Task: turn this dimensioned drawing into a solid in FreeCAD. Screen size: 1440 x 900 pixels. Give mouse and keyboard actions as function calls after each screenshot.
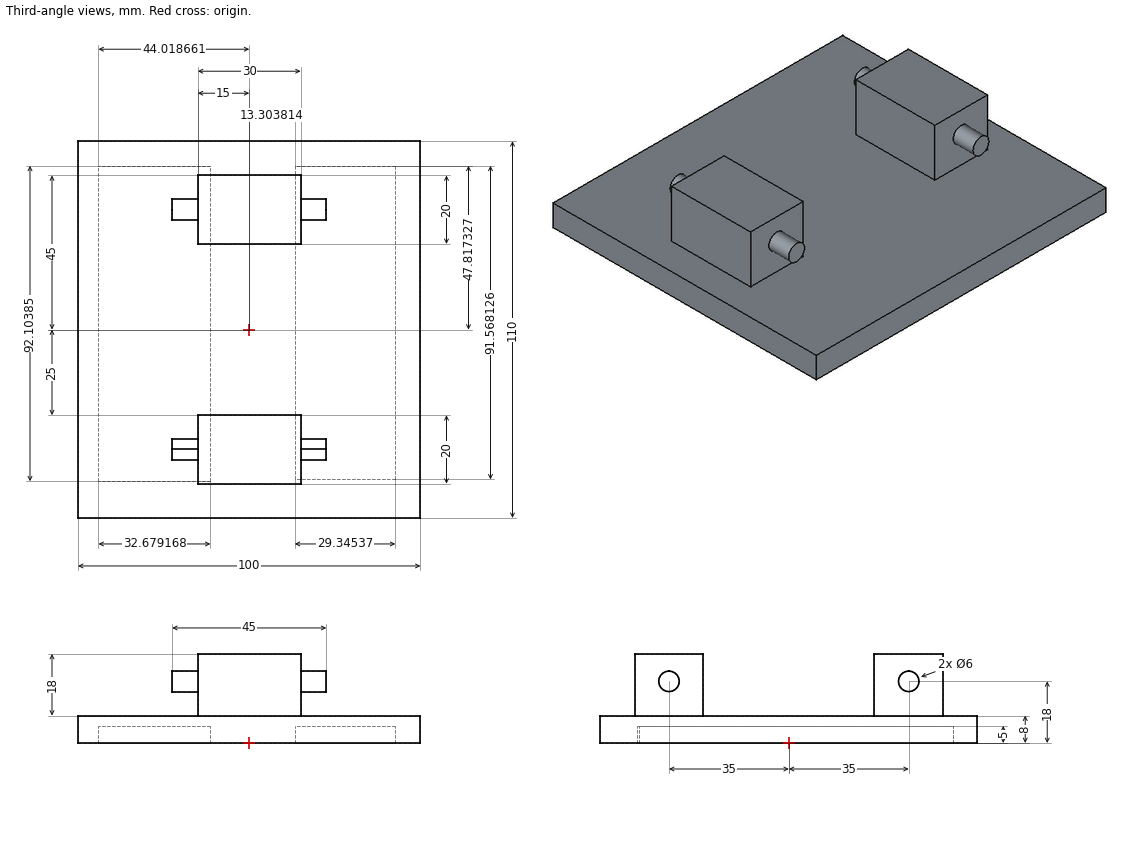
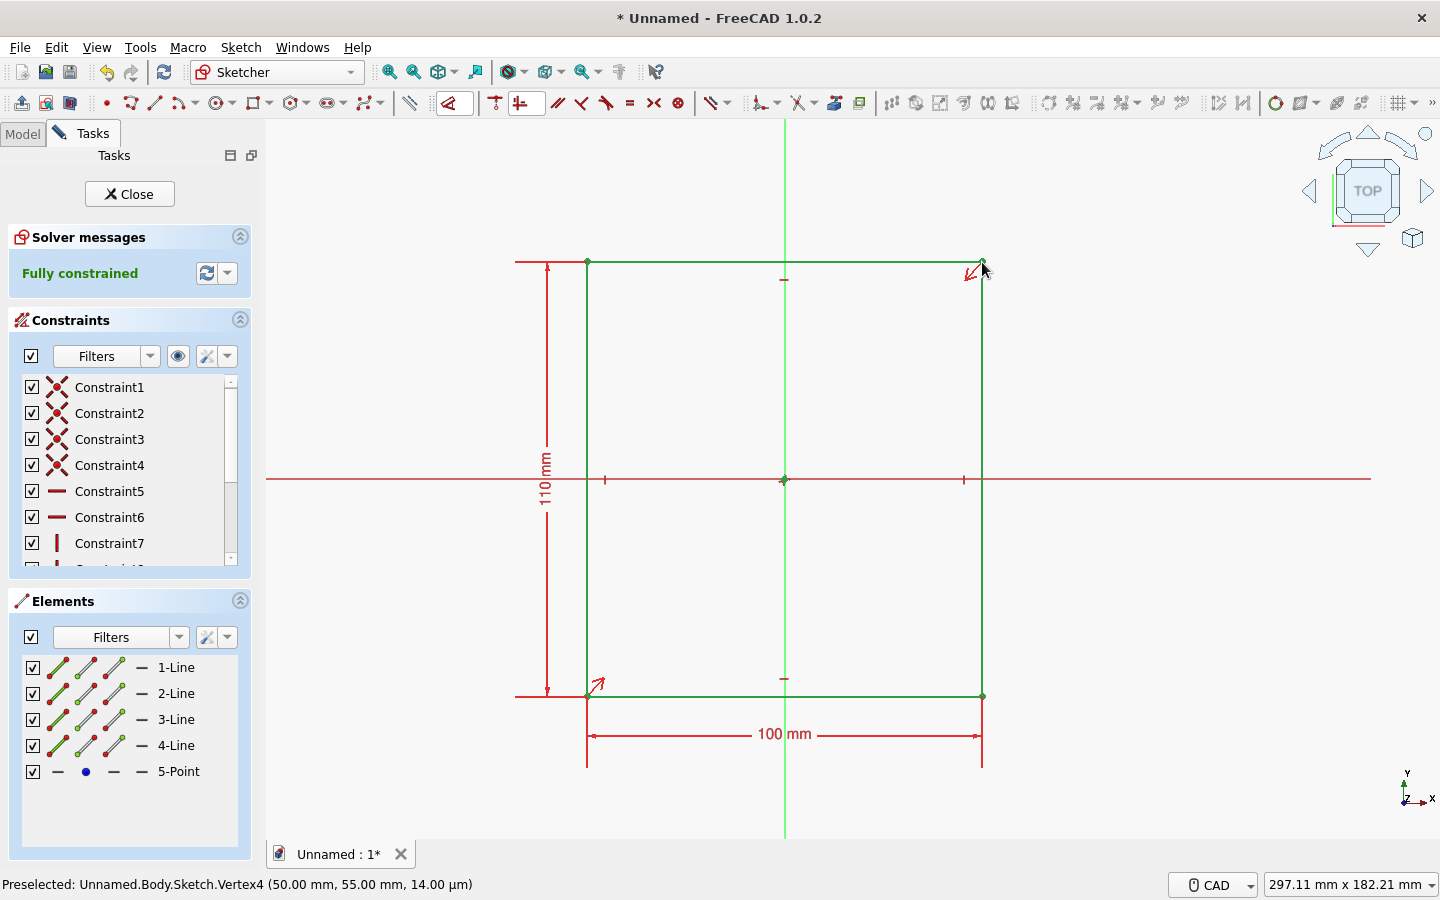
click(130, 194)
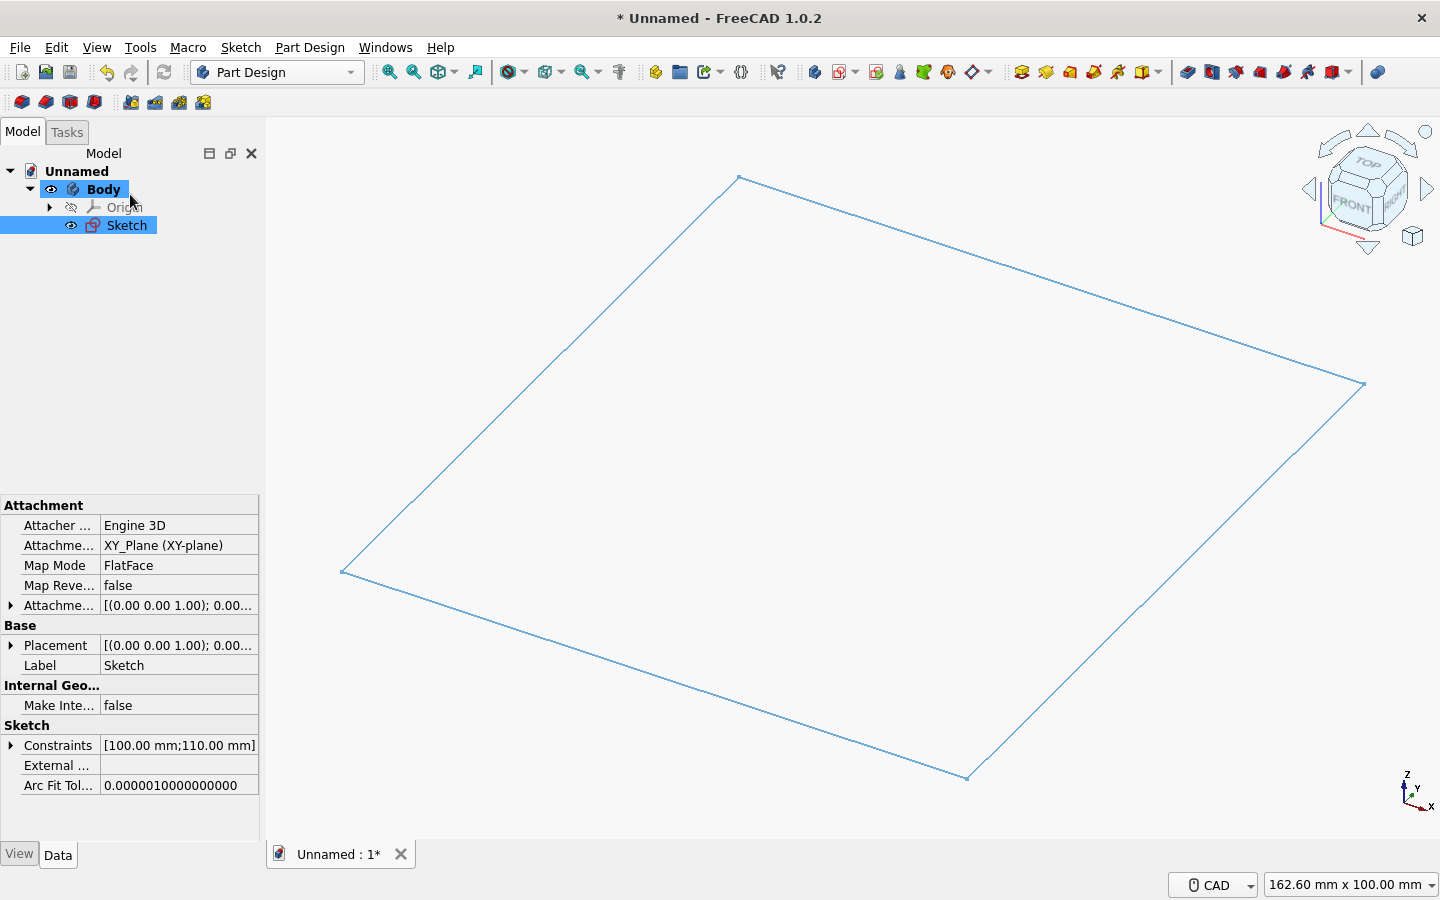
click(1022, 72)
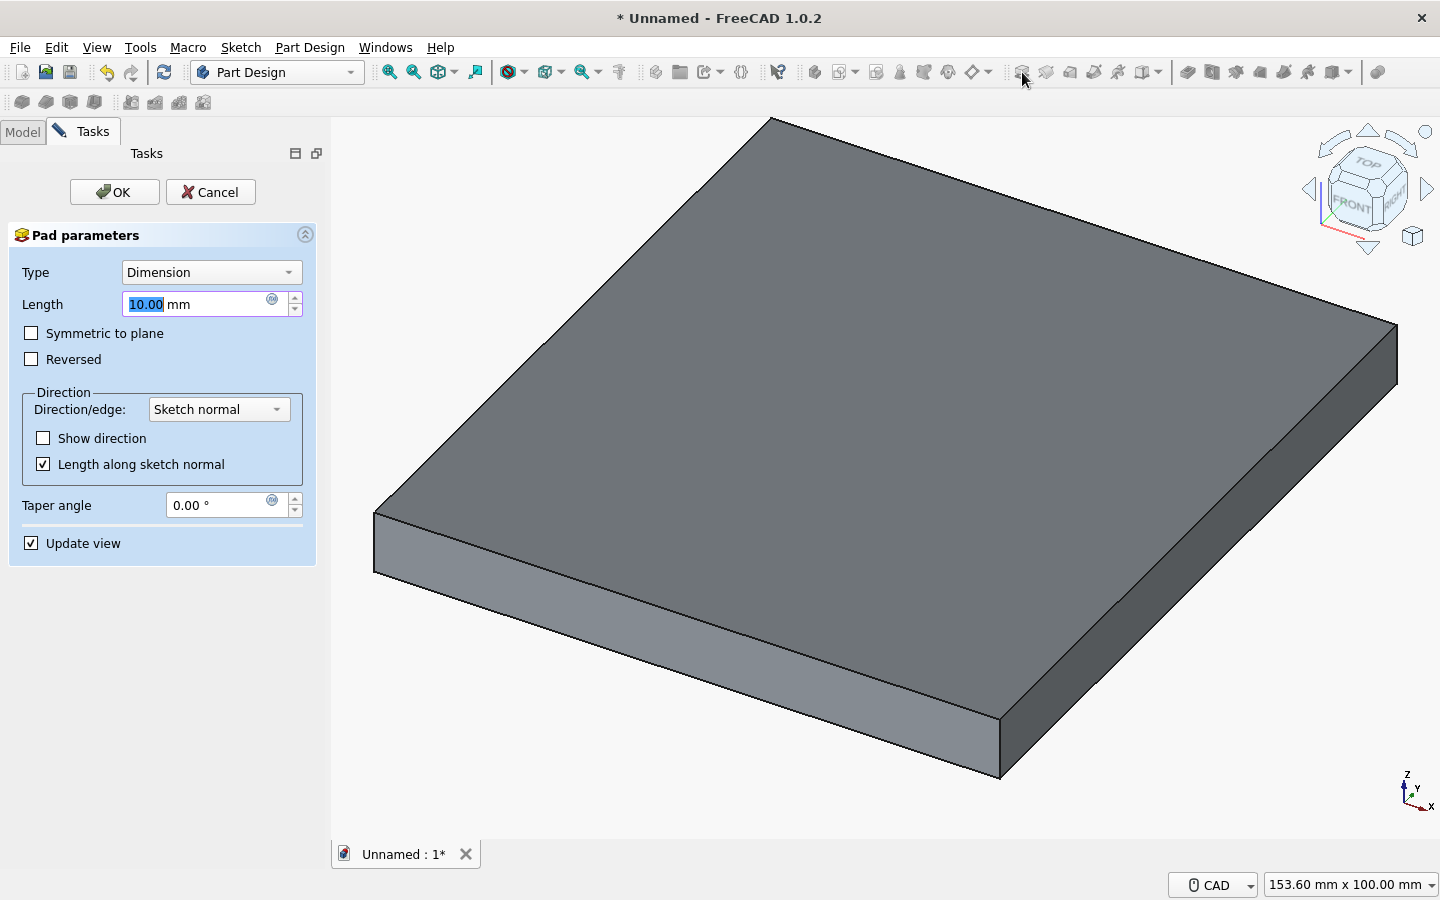
text(8)
key(Tab)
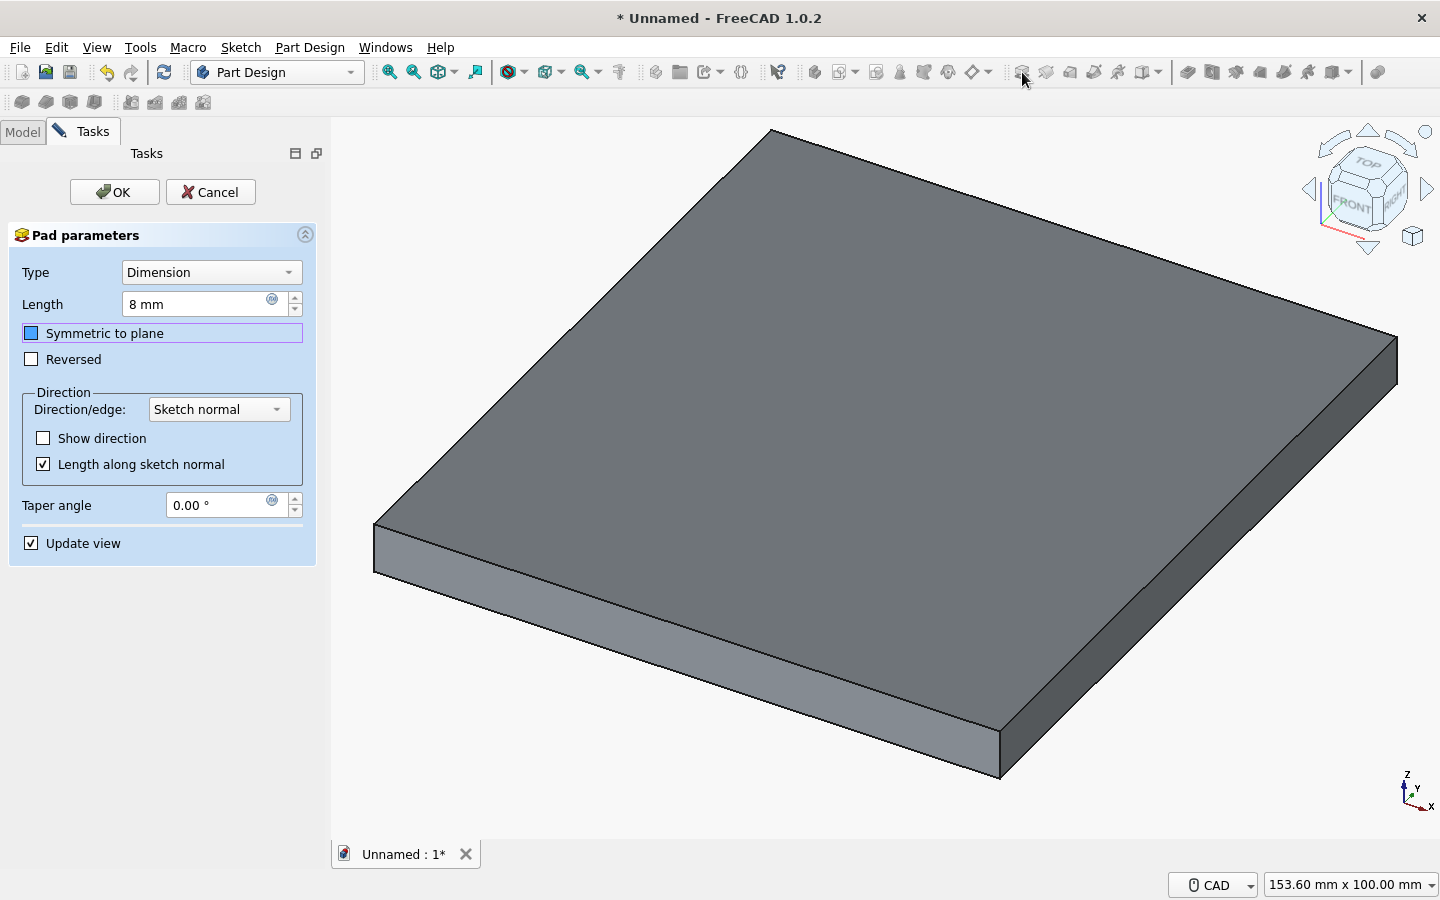
click(115, 192)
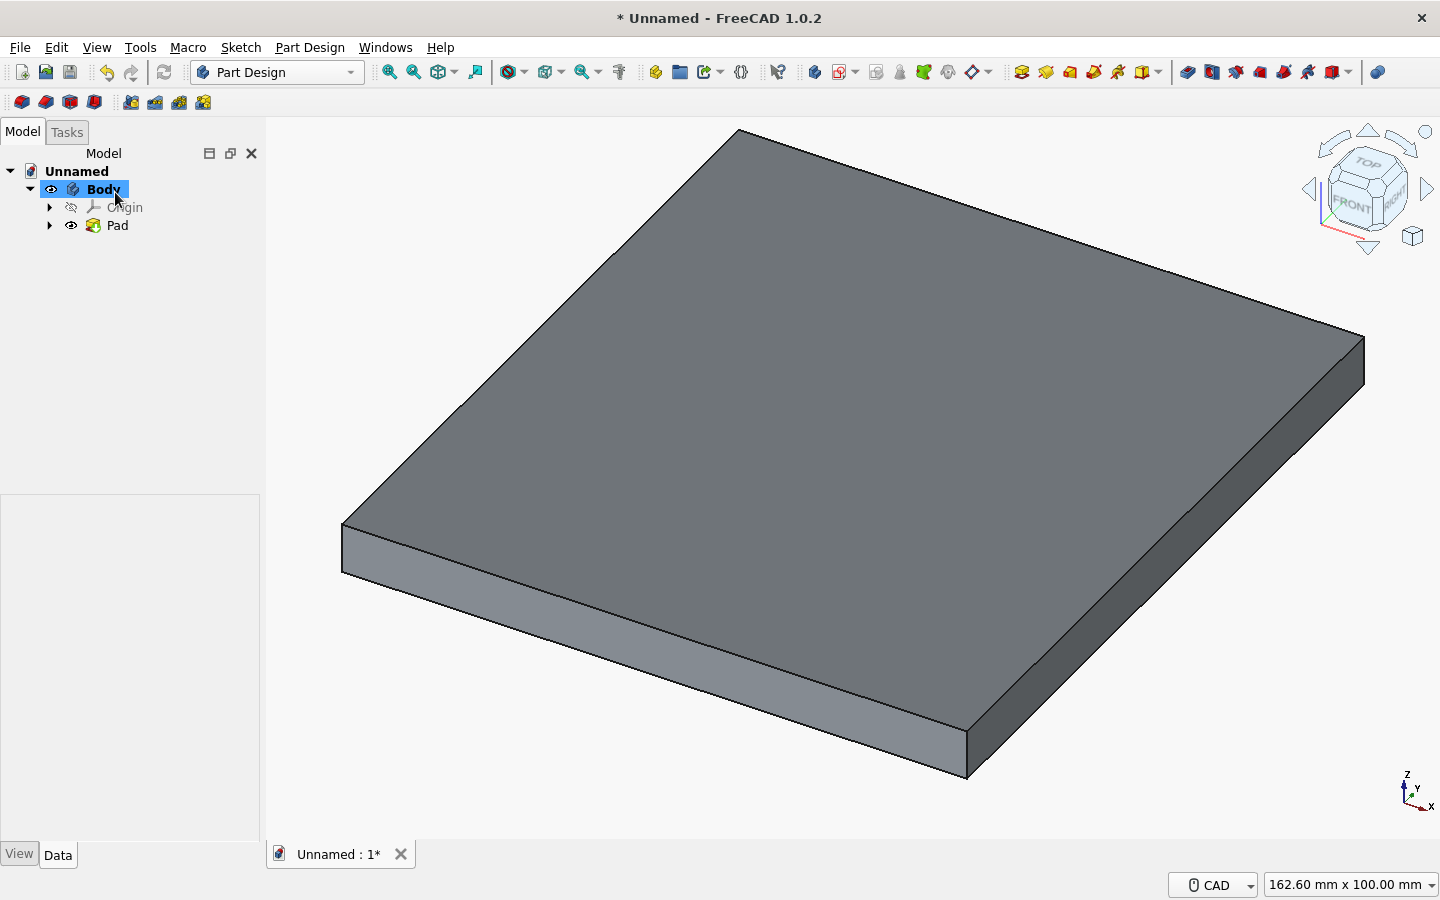
click(853, 430)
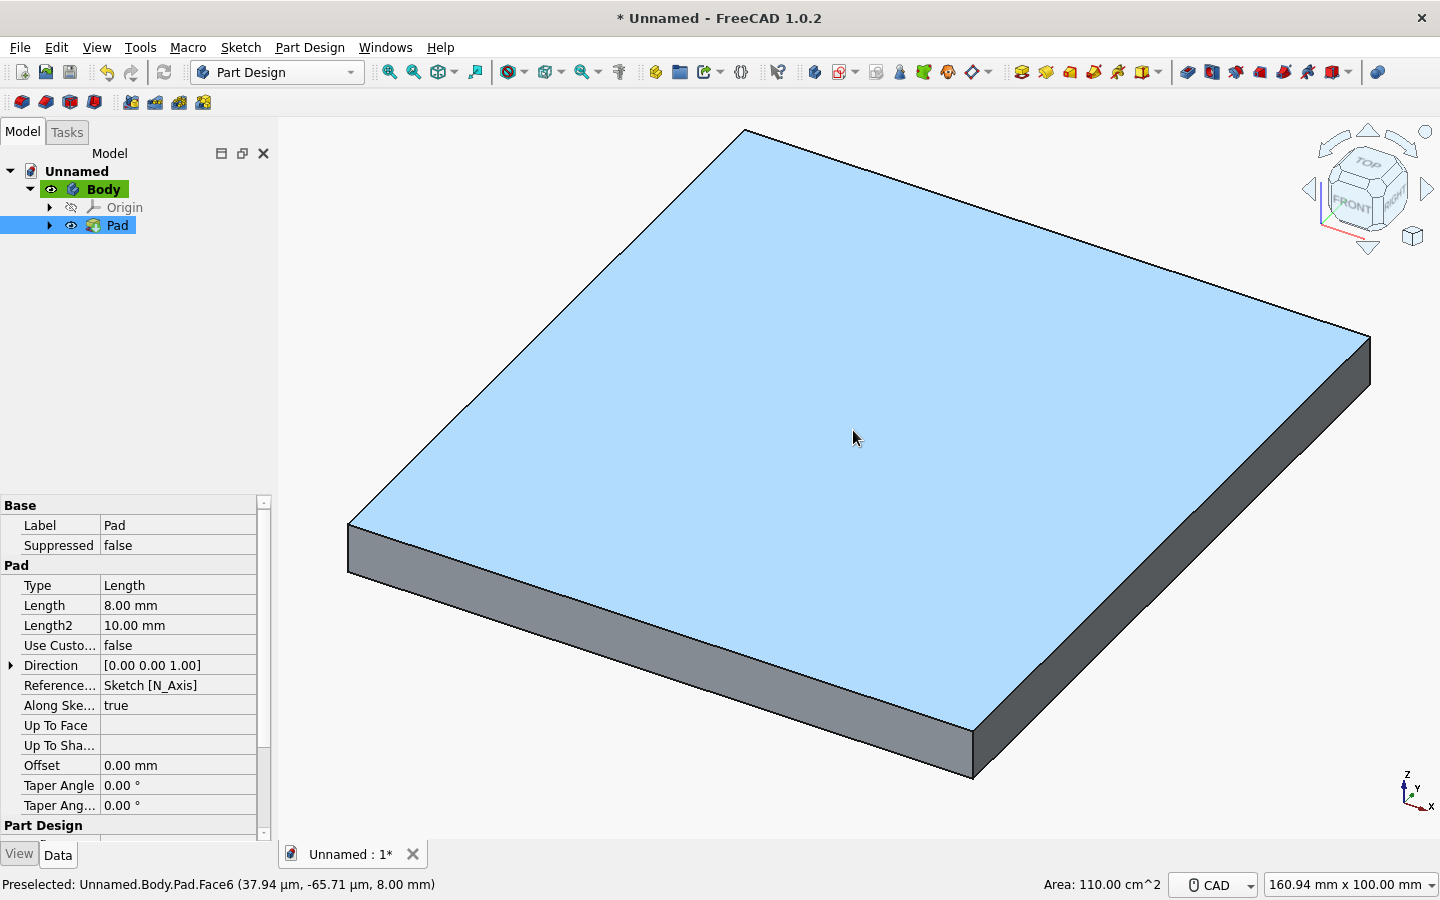
click(840, 72)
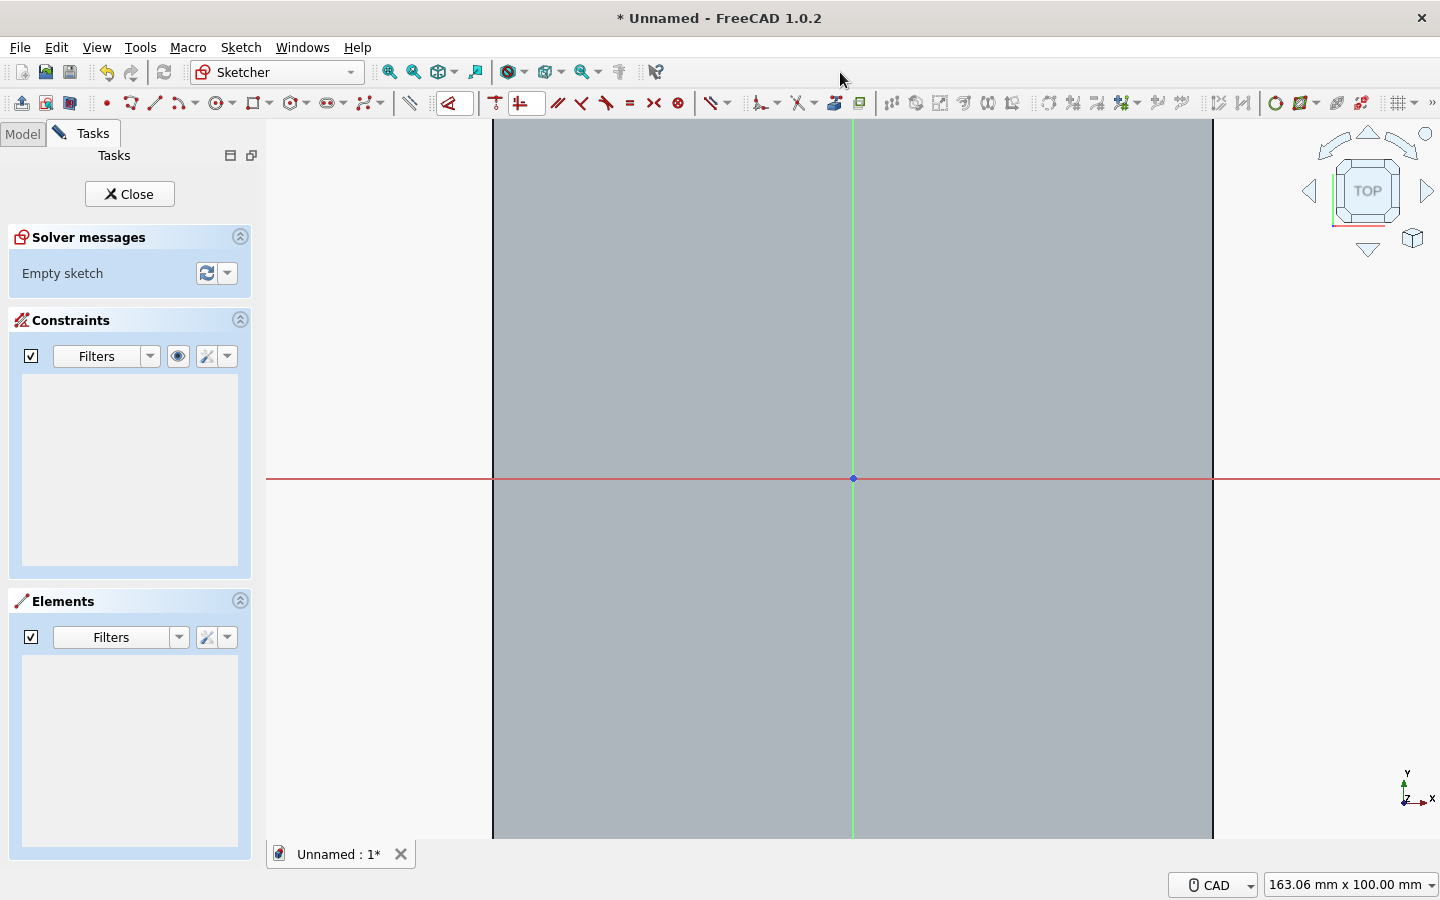
scroll(645, 479, down, 2)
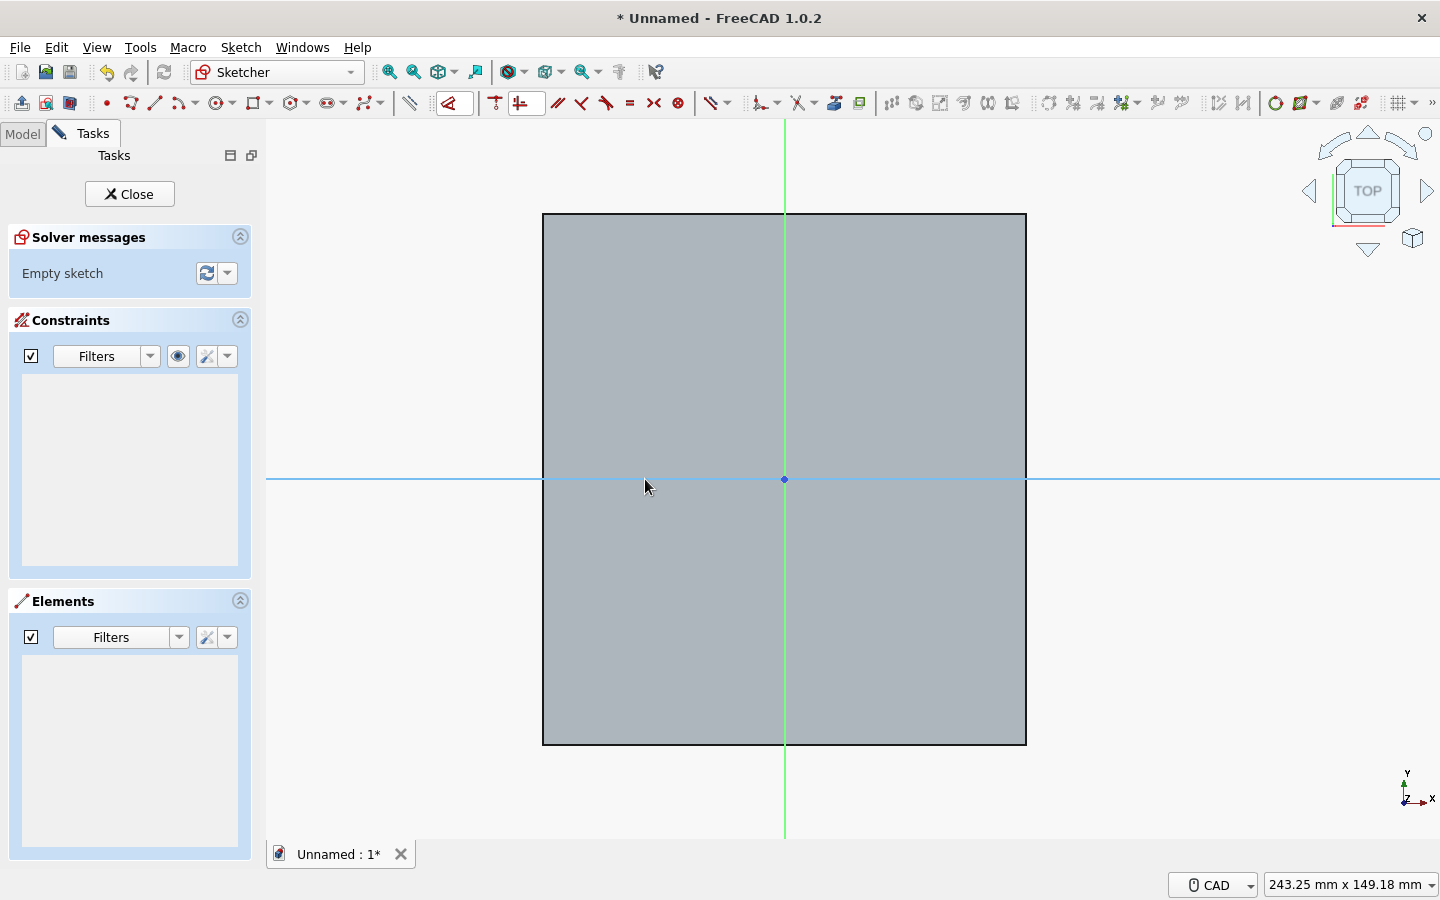
key(g)
key(r)